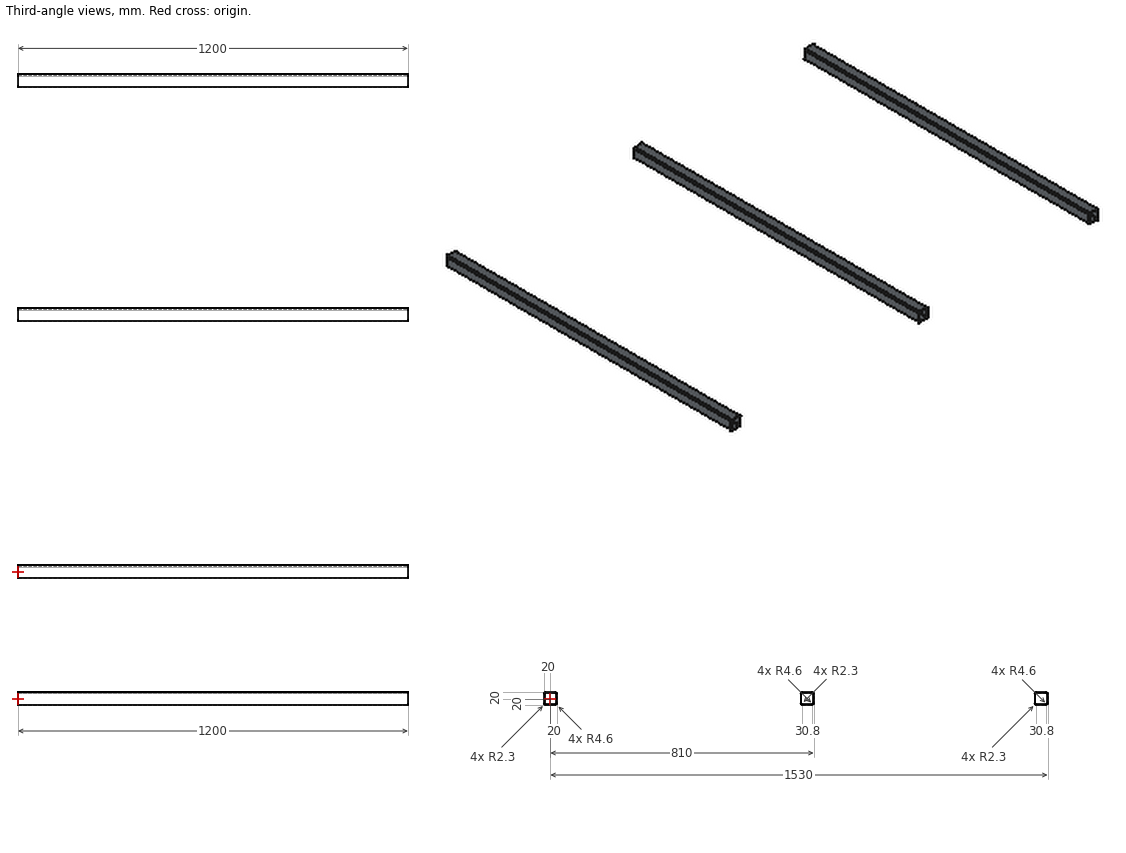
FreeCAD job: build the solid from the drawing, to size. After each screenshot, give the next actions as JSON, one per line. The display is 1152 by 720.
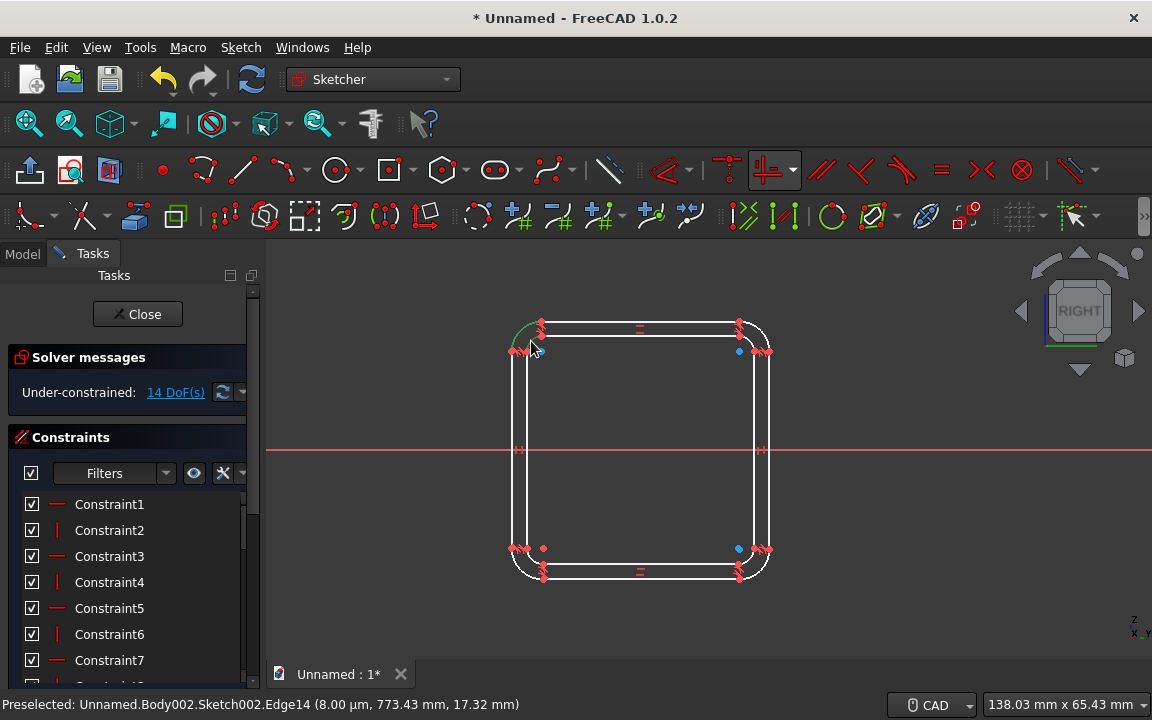
{"action": "left_click", "coordinate": [728, 170]}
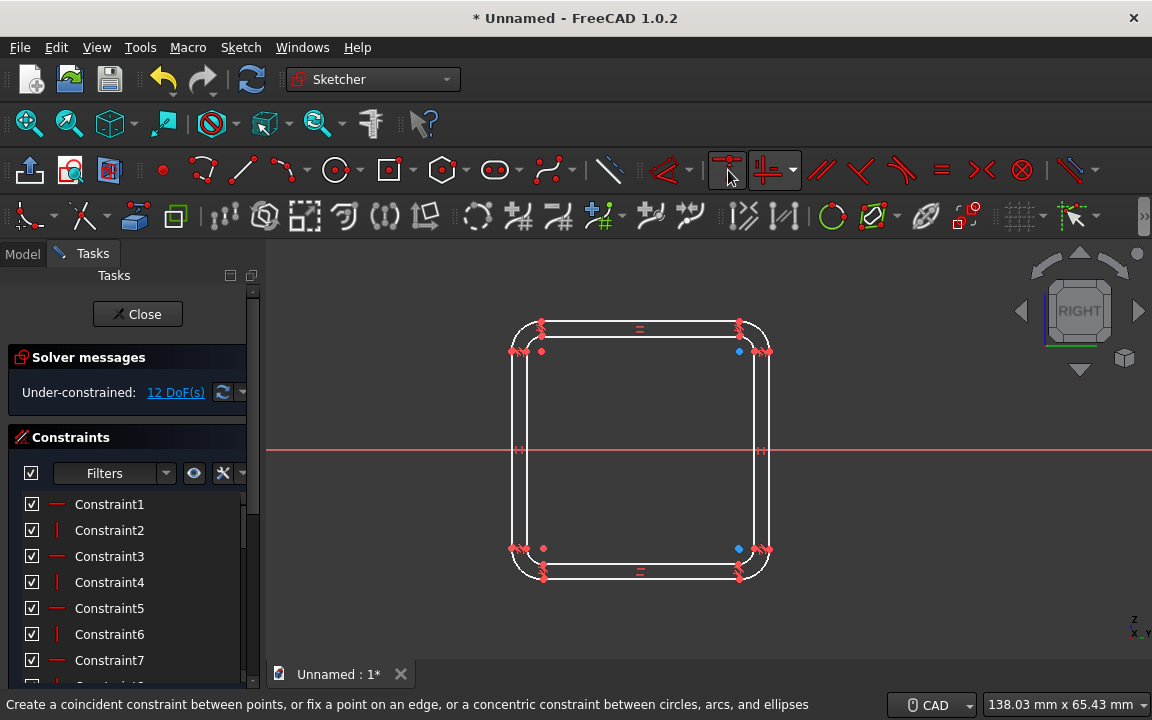
{"action": "left_click", "coordinate": [766, 338]}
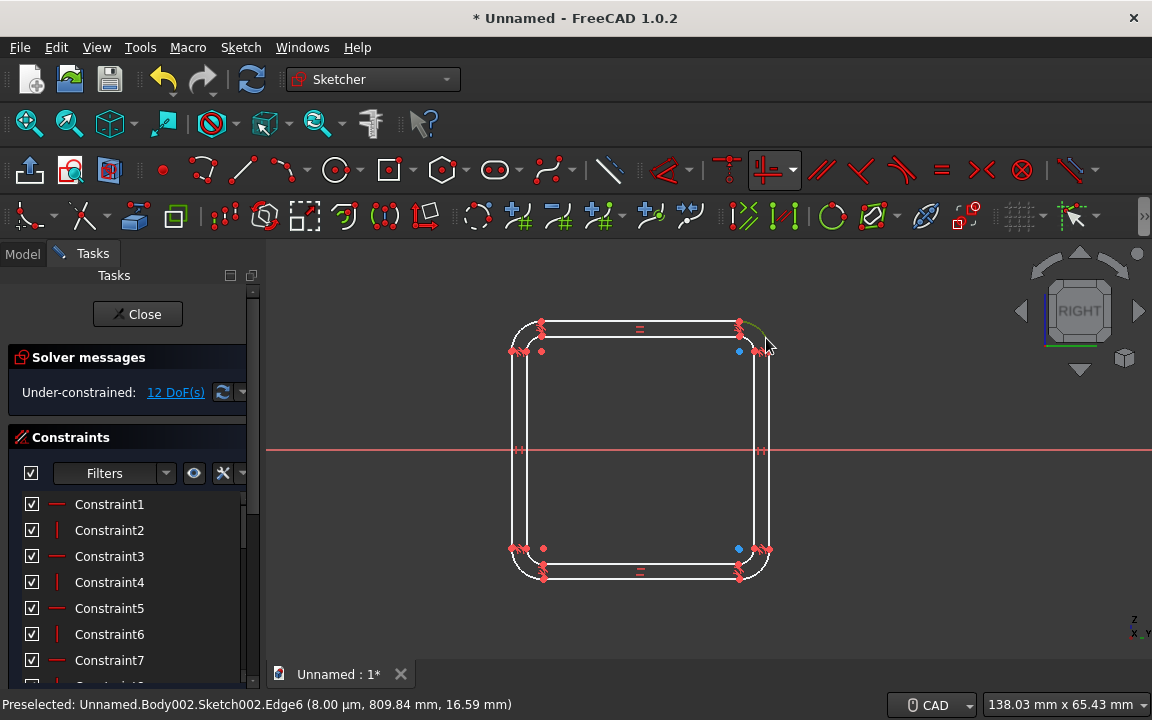
{"action": "left_click", "coordinate": [750, 341]}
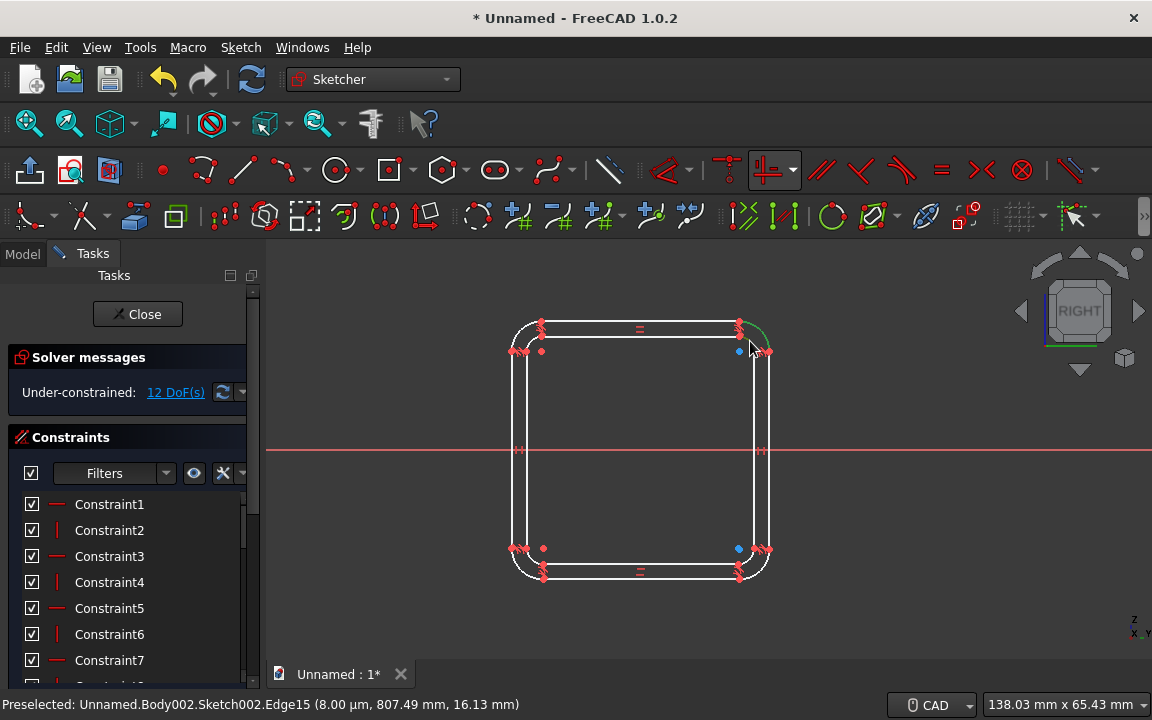
{"action": "key", "text": "c"}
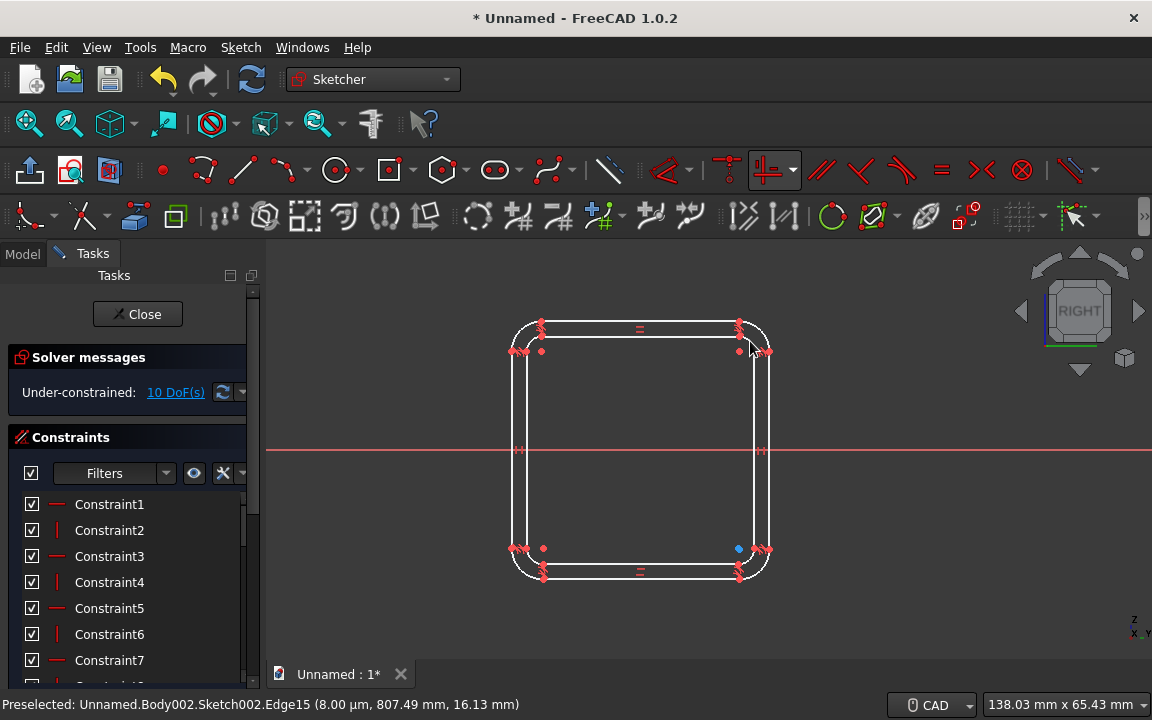
{"action": "left_click", "coordinate": [753, 576]}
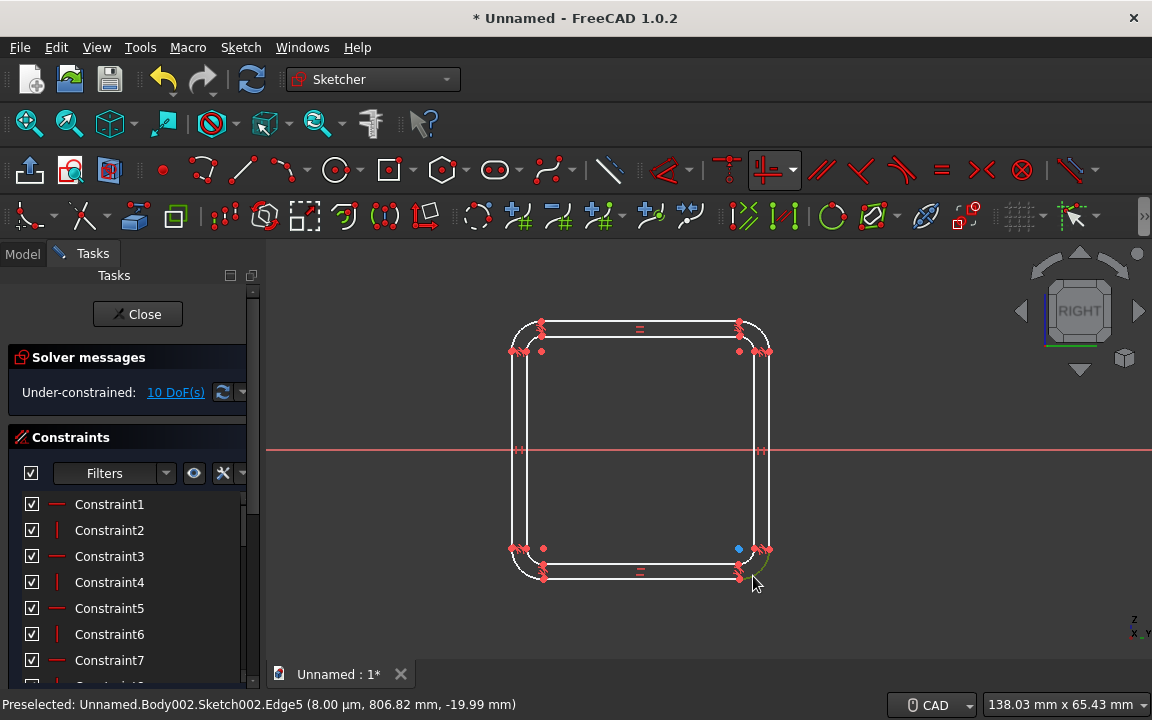
{"action": "left_click", "coordinate": [766, 338]}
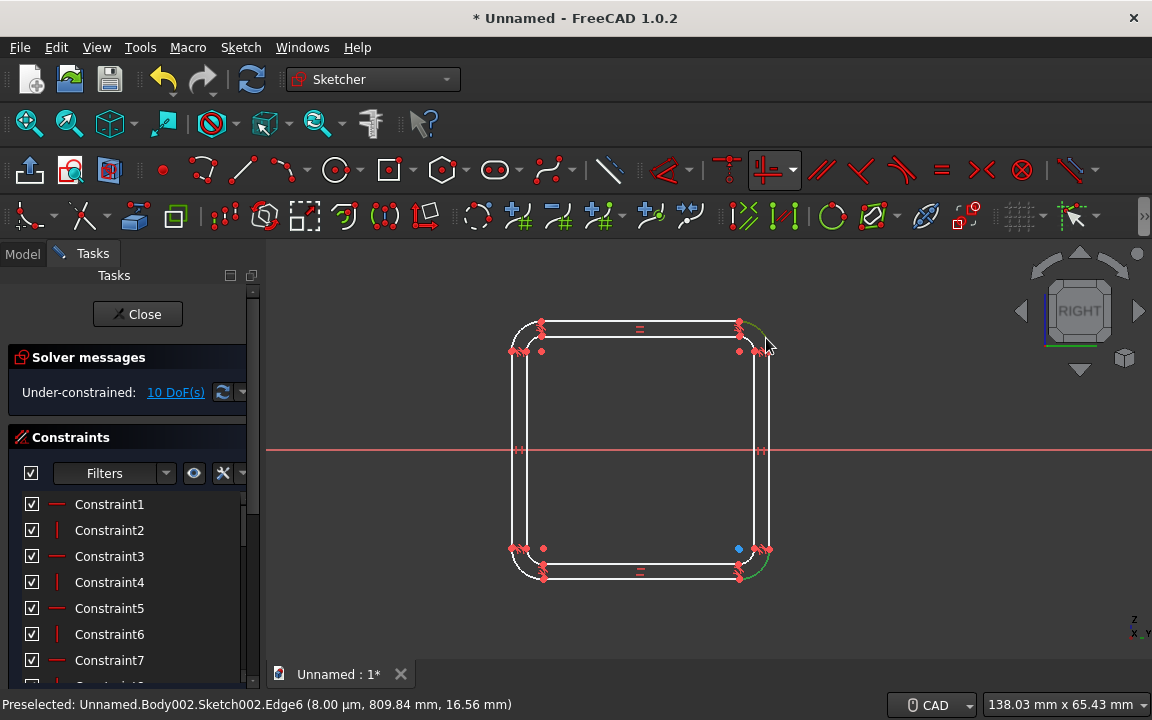
{"action": "left_click", "coordinate": [528, 325]}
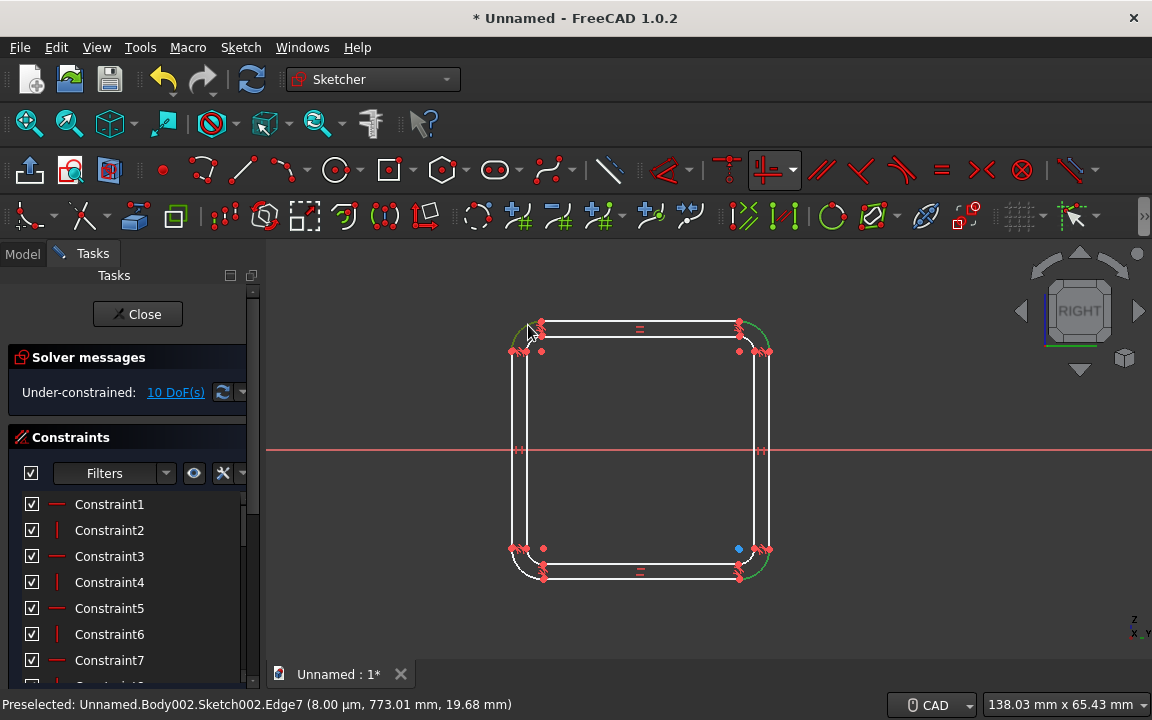
{"action": "left_click", "coordinate": [515, 562]}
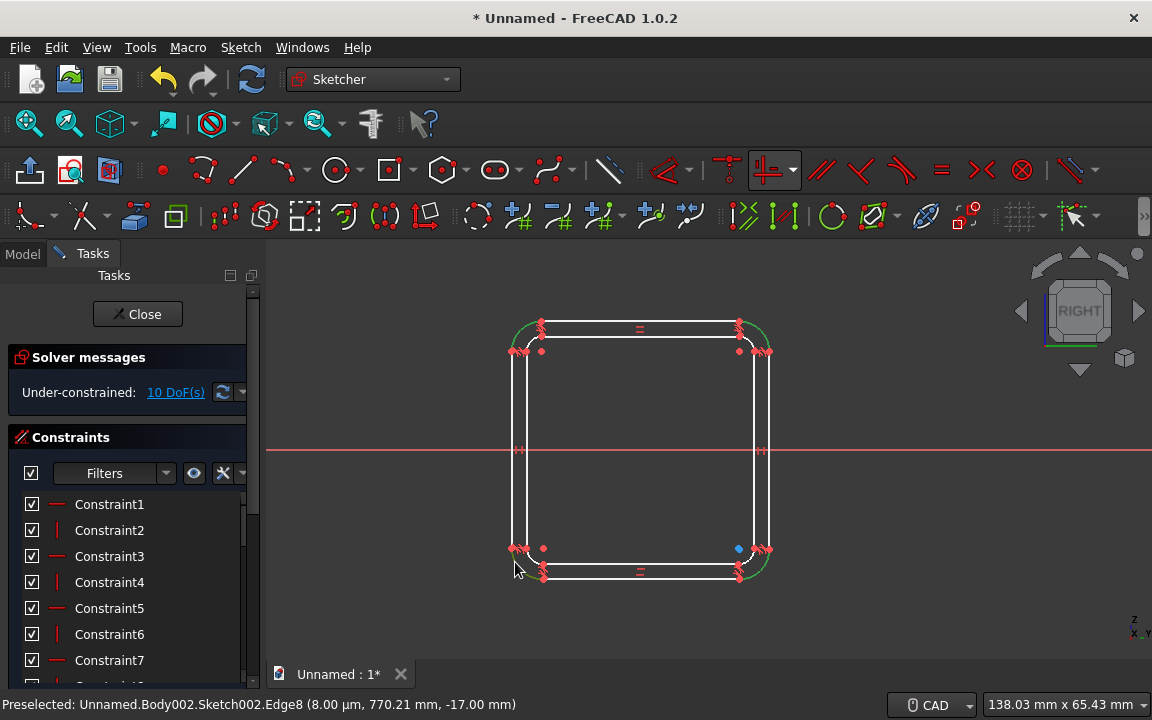
{"action": "left_click", "coordinate": [942, 170]}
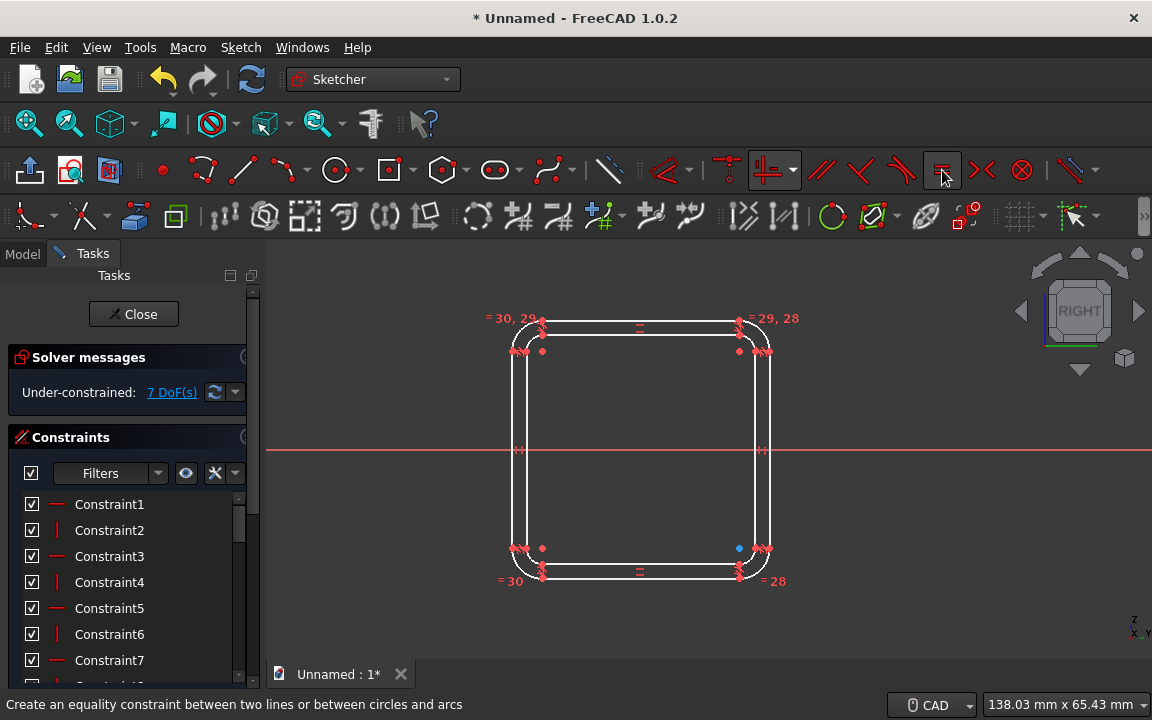
{"action": "left_click", "coordinate": [531, 560]}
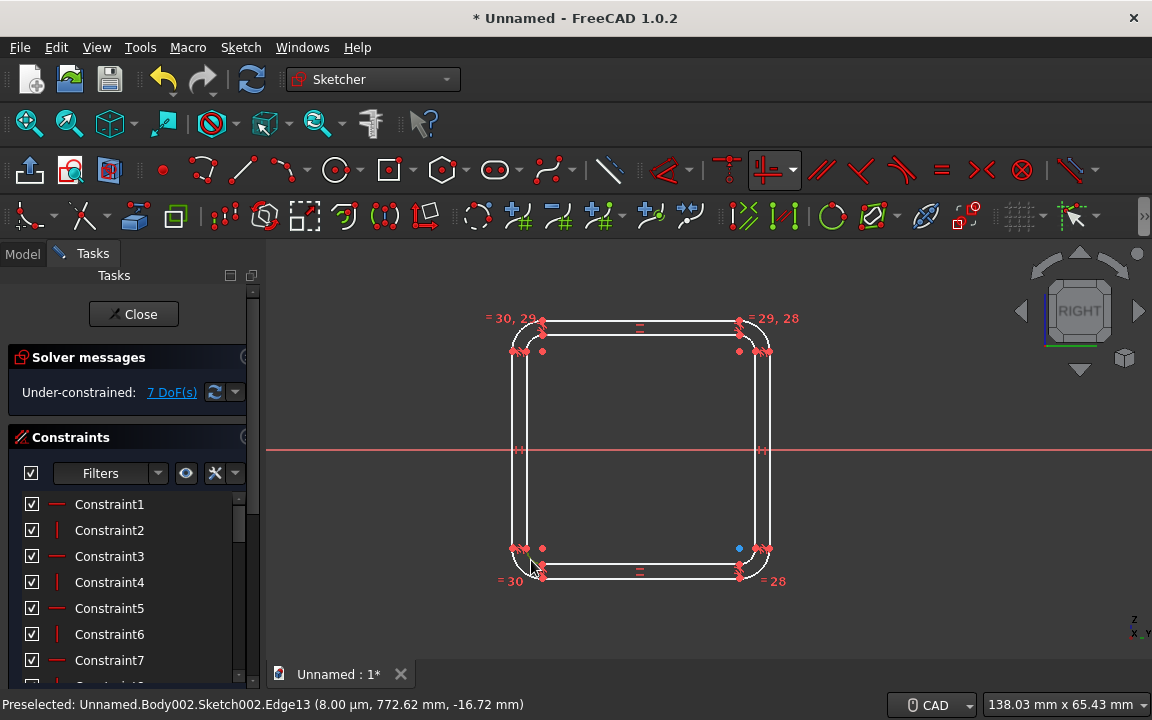
{"action": "left_click", "coordinate": [750, 560]}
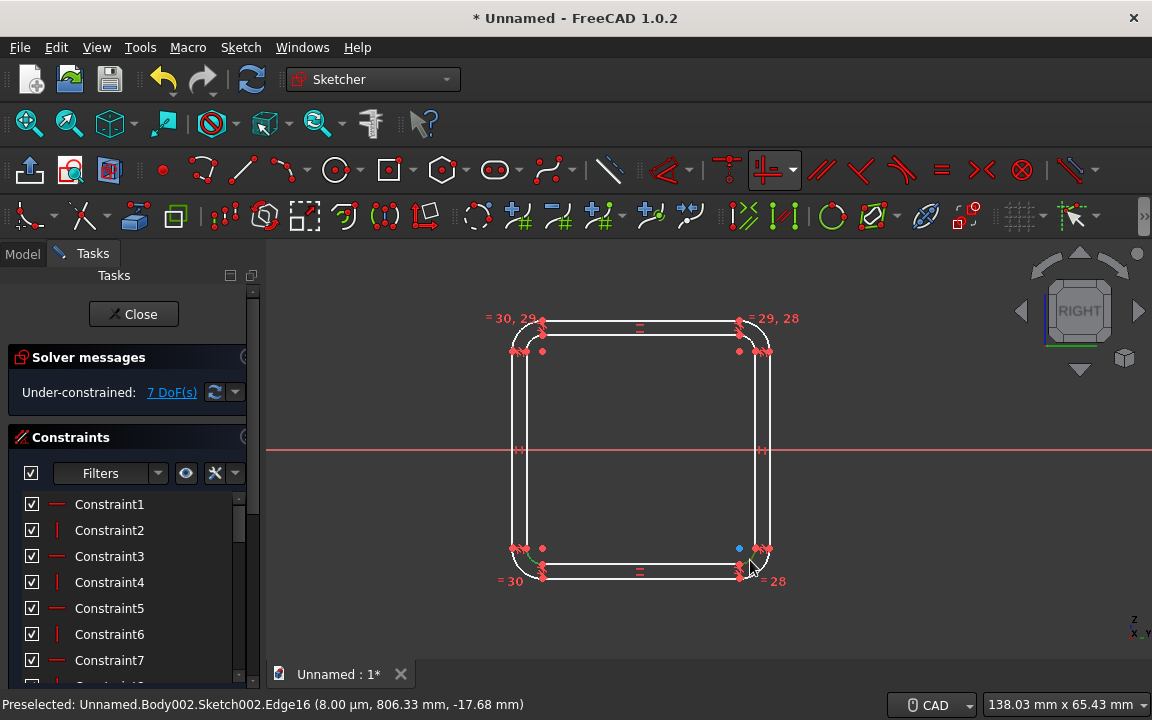
{"action": "key", "text": "e"}